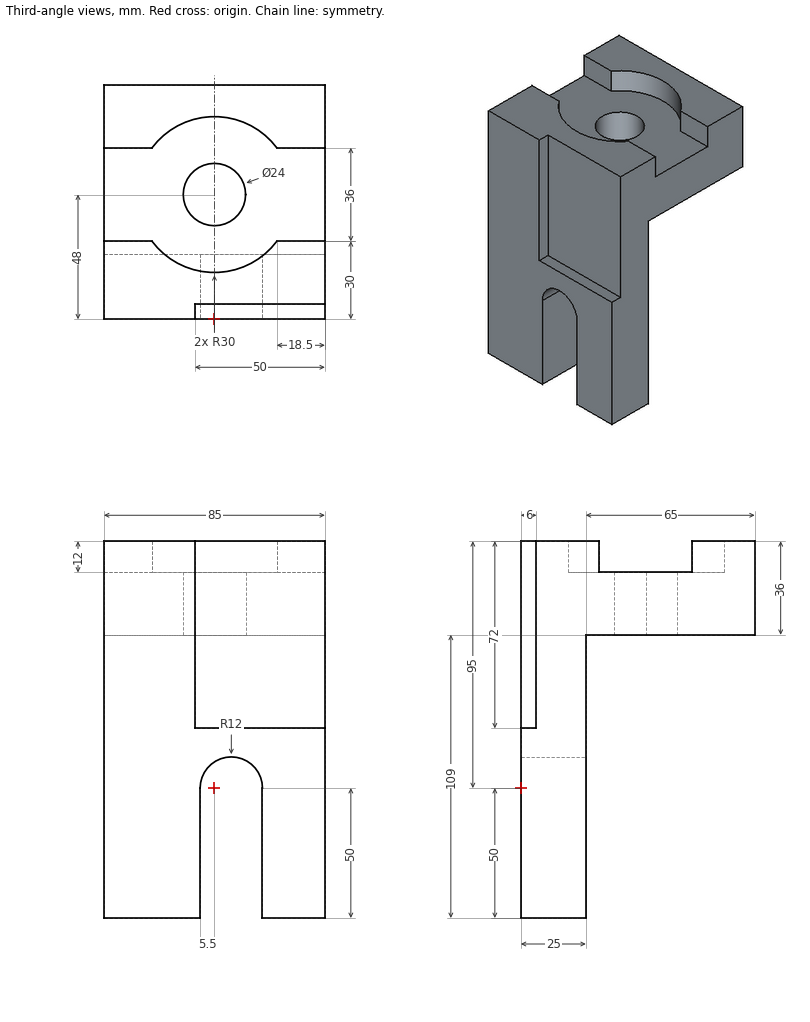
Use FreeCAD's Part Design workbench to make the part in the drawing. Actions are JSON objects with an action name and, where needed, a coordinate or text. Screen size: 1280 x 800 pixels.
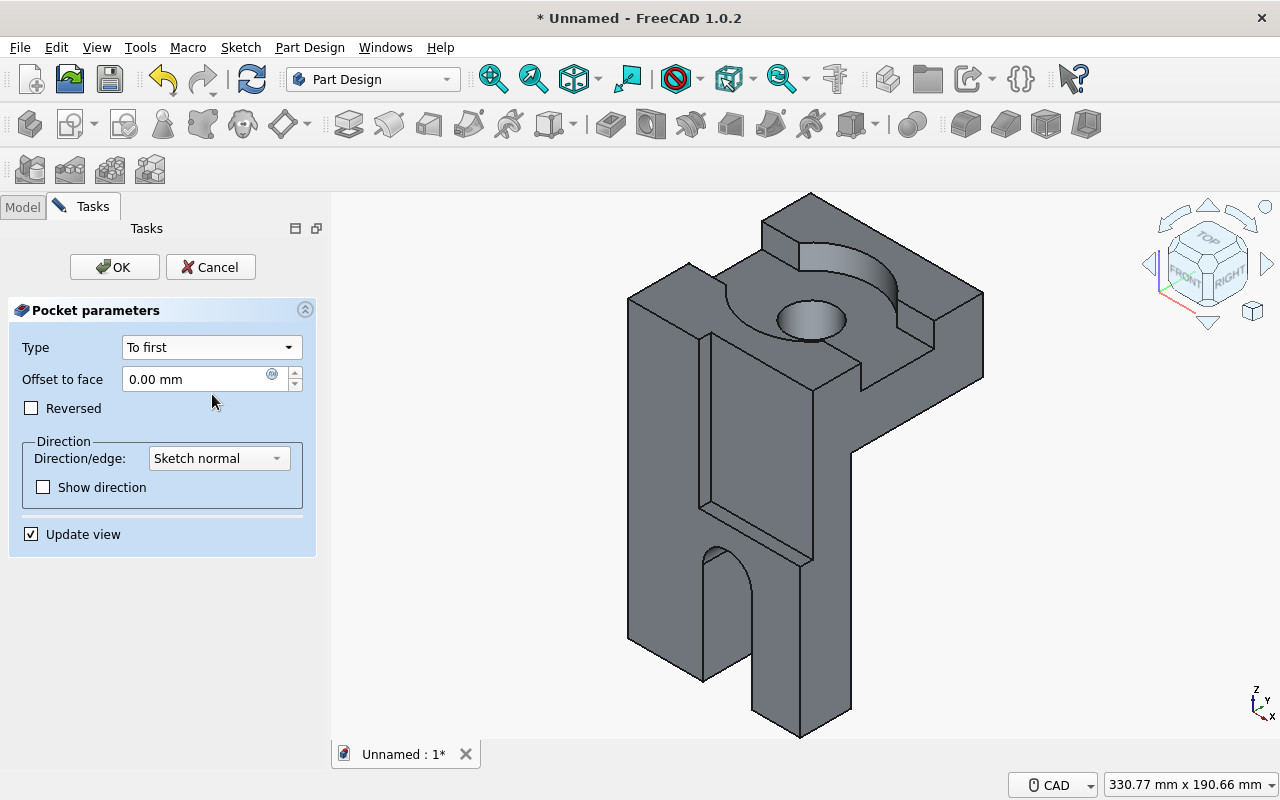
{"action": "left_click", "coordinate": [115, 267]}